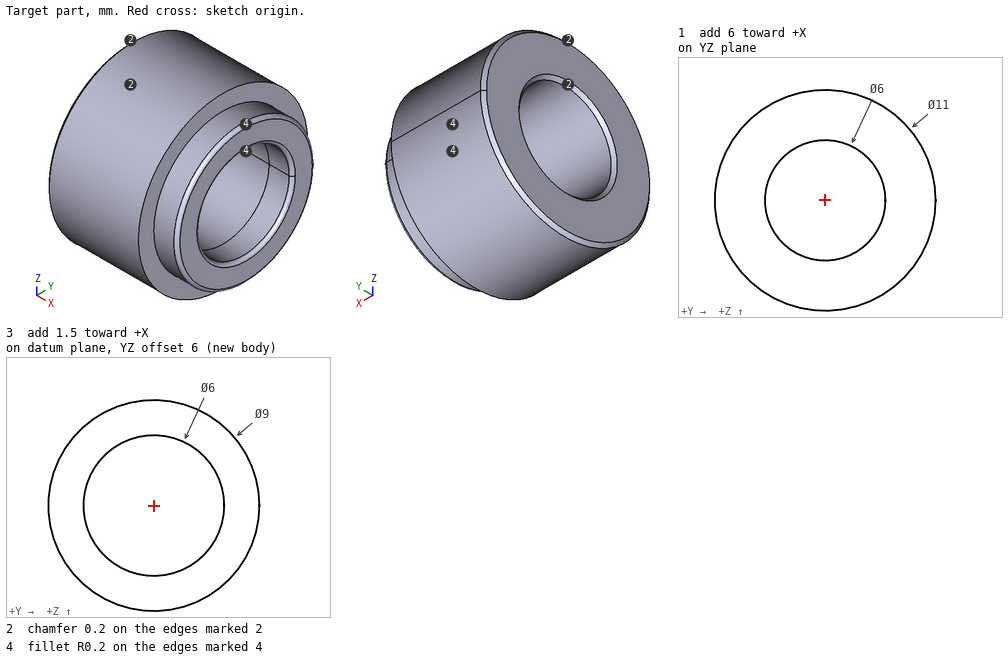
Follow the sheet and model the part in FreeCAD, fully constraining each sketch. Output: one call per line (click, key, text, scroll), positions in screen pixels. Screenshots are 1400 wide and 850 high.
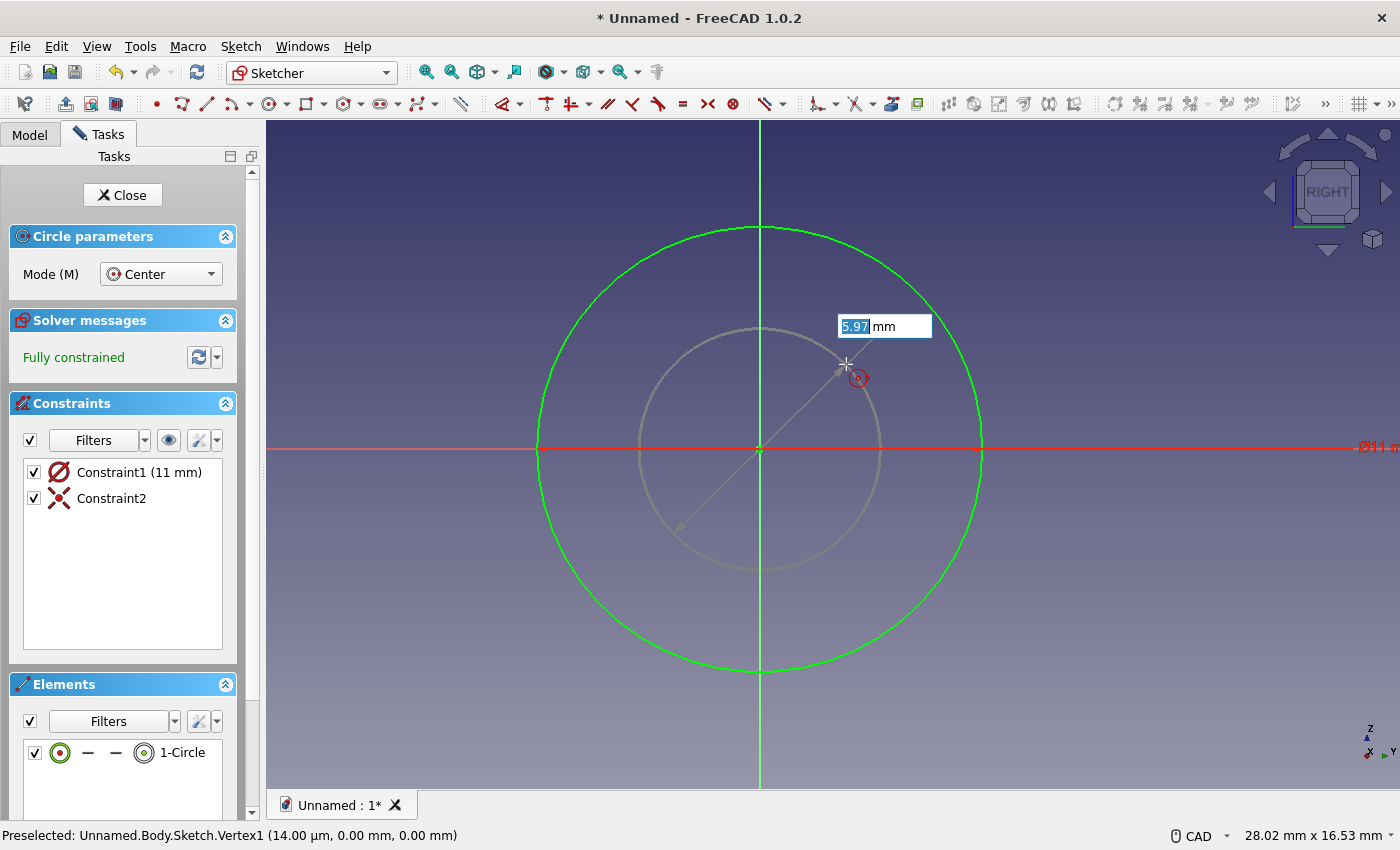
text(6)
key(Return)
key(Escape)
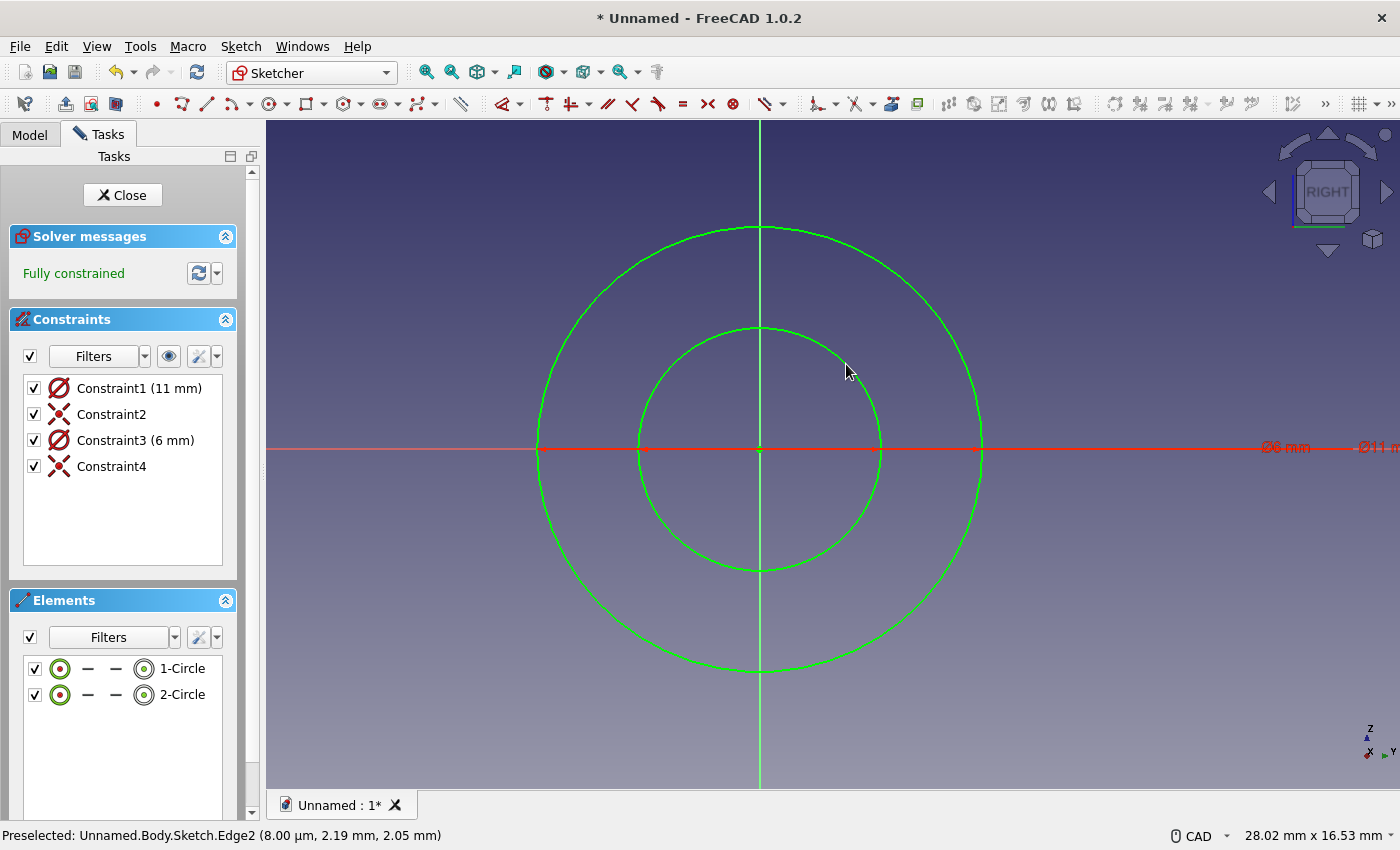
click(123, 195)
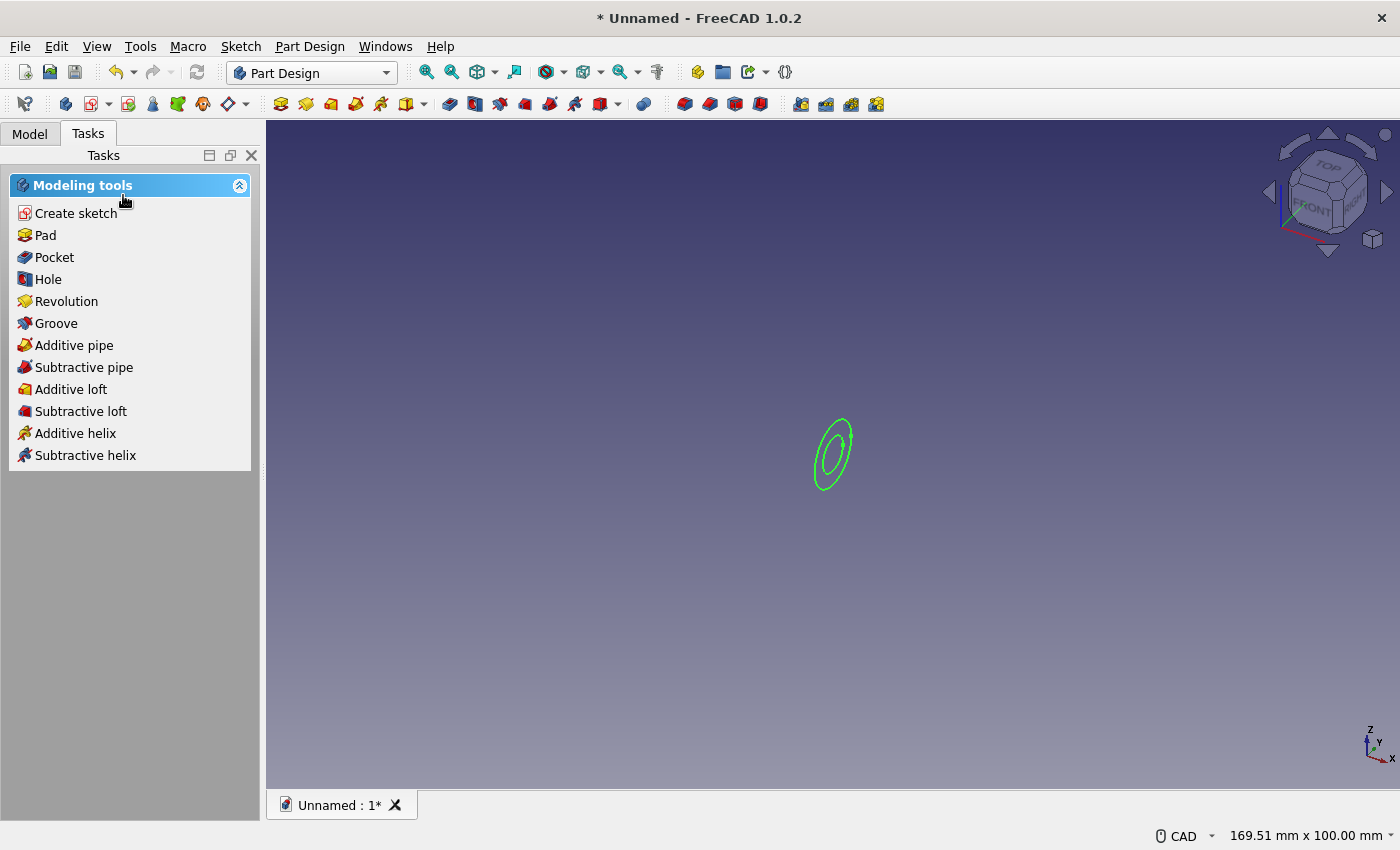
click(281, 104)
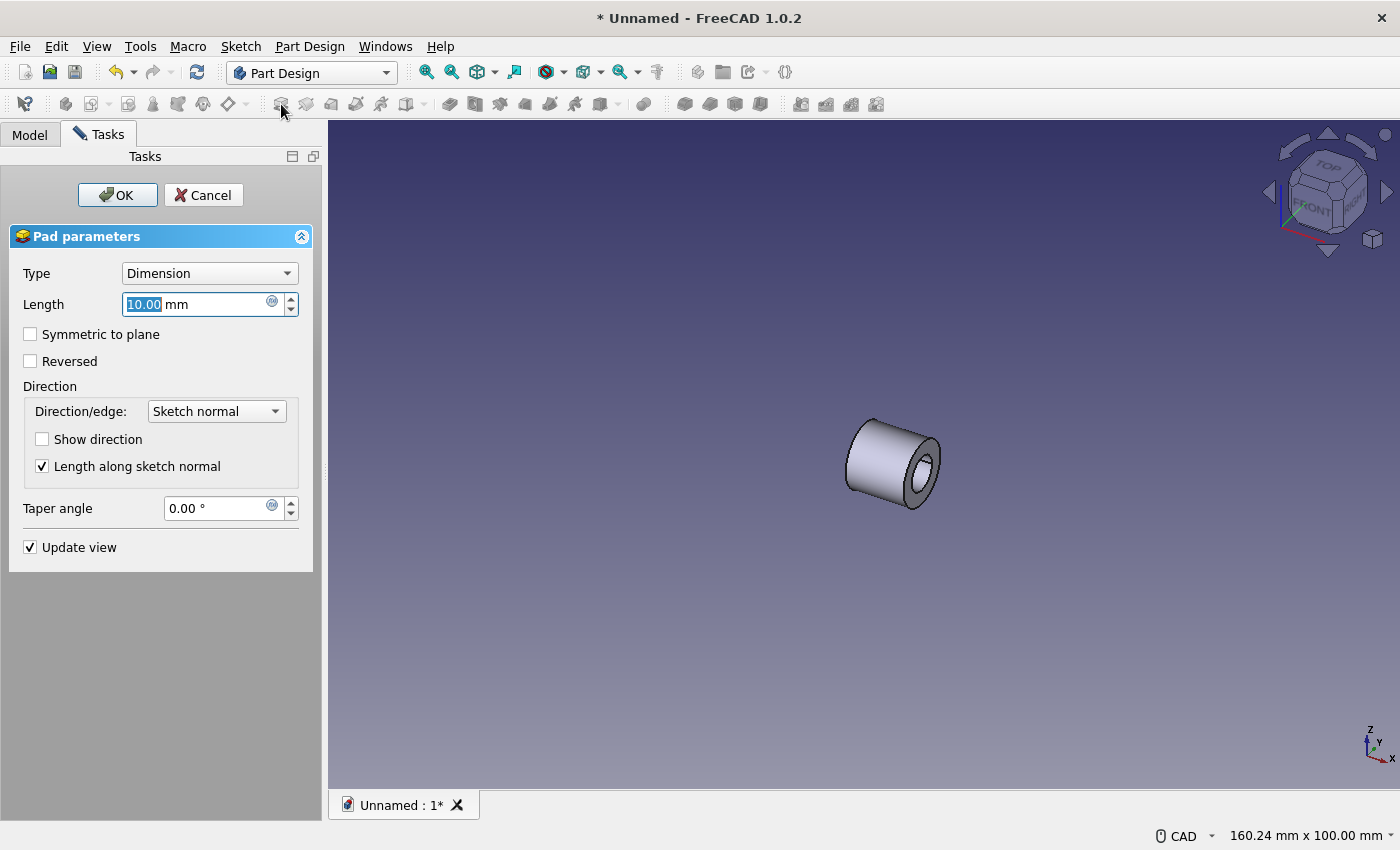
text(6)
key(Tab)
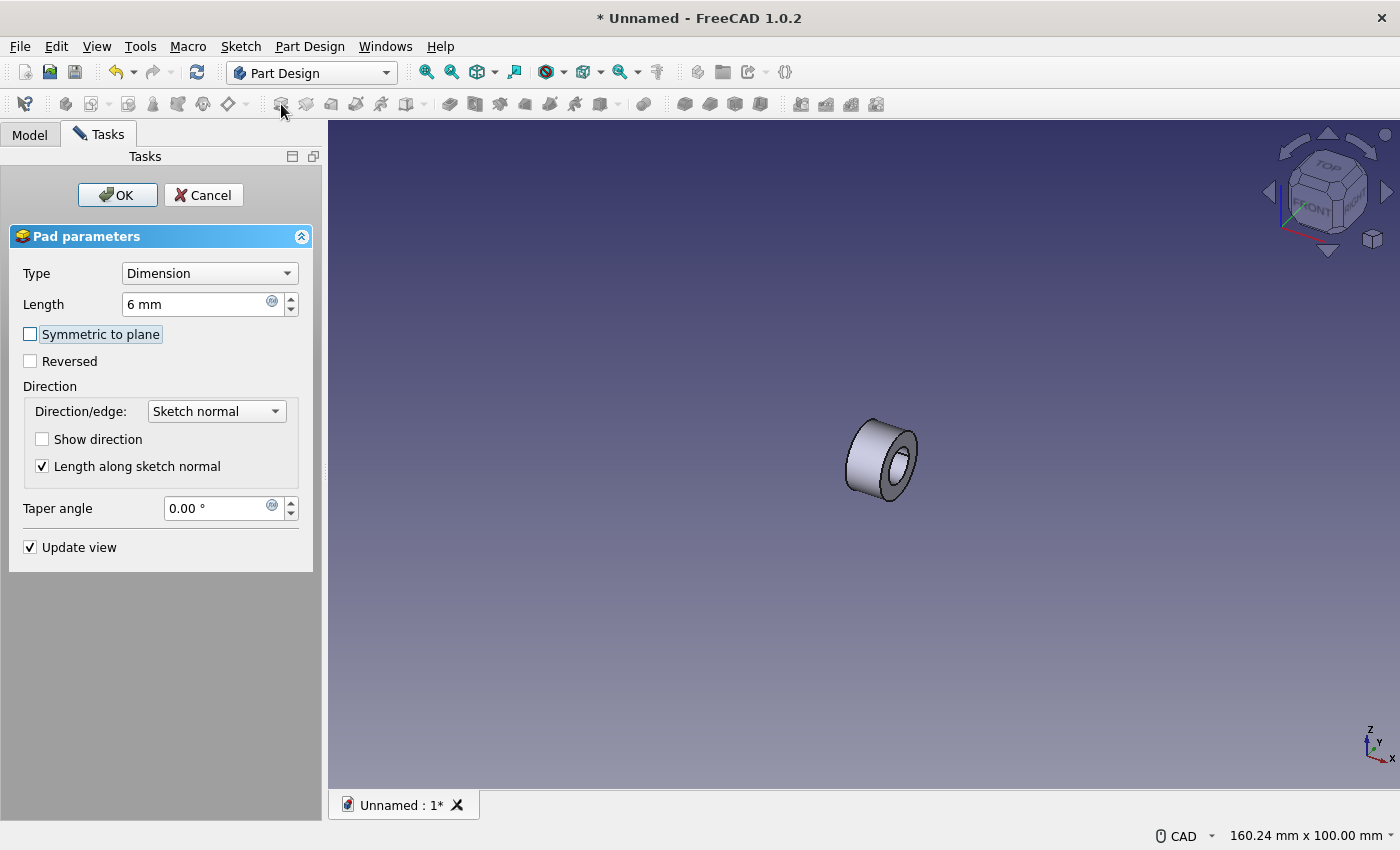
click(118, 195)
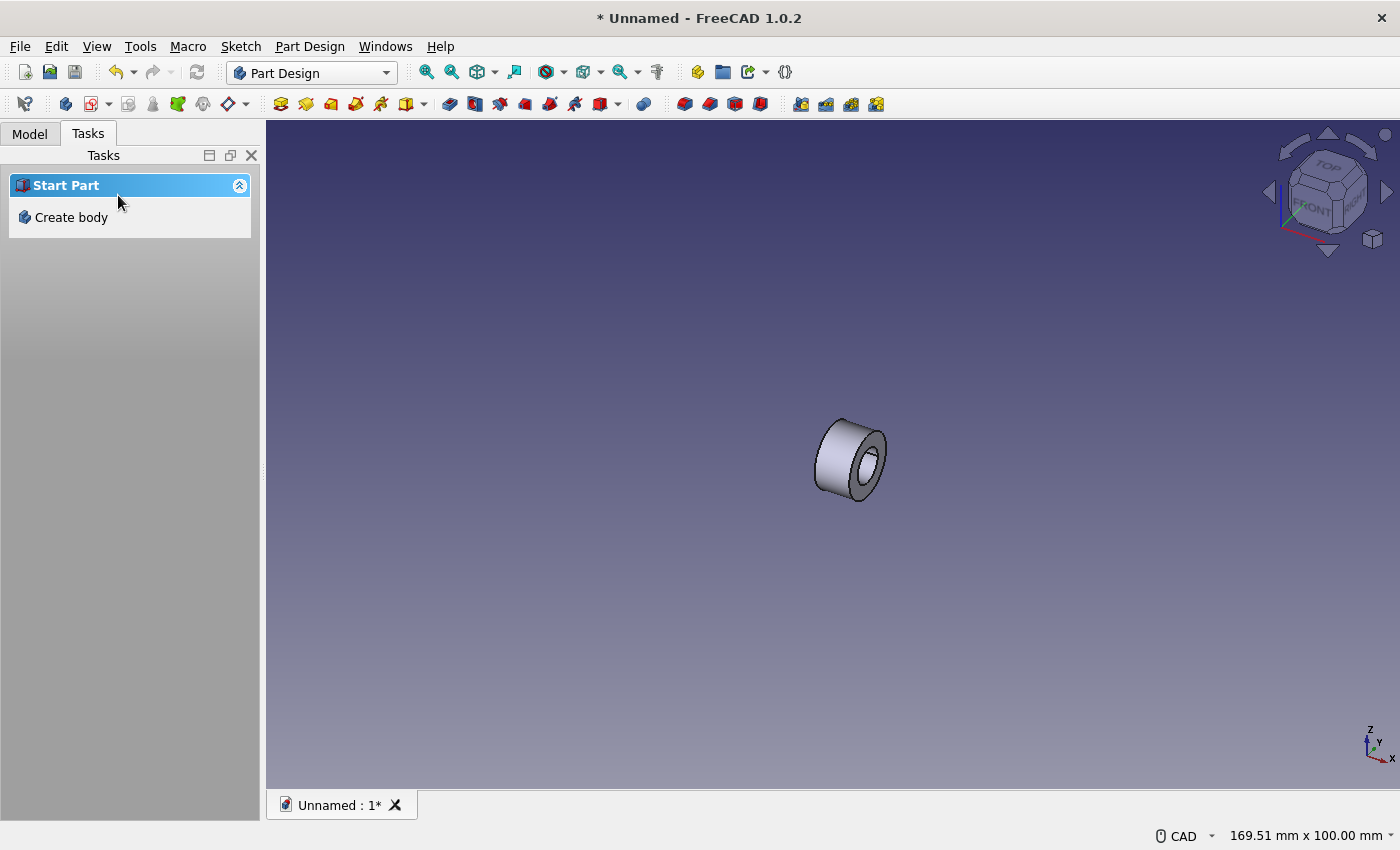
click(427, 72)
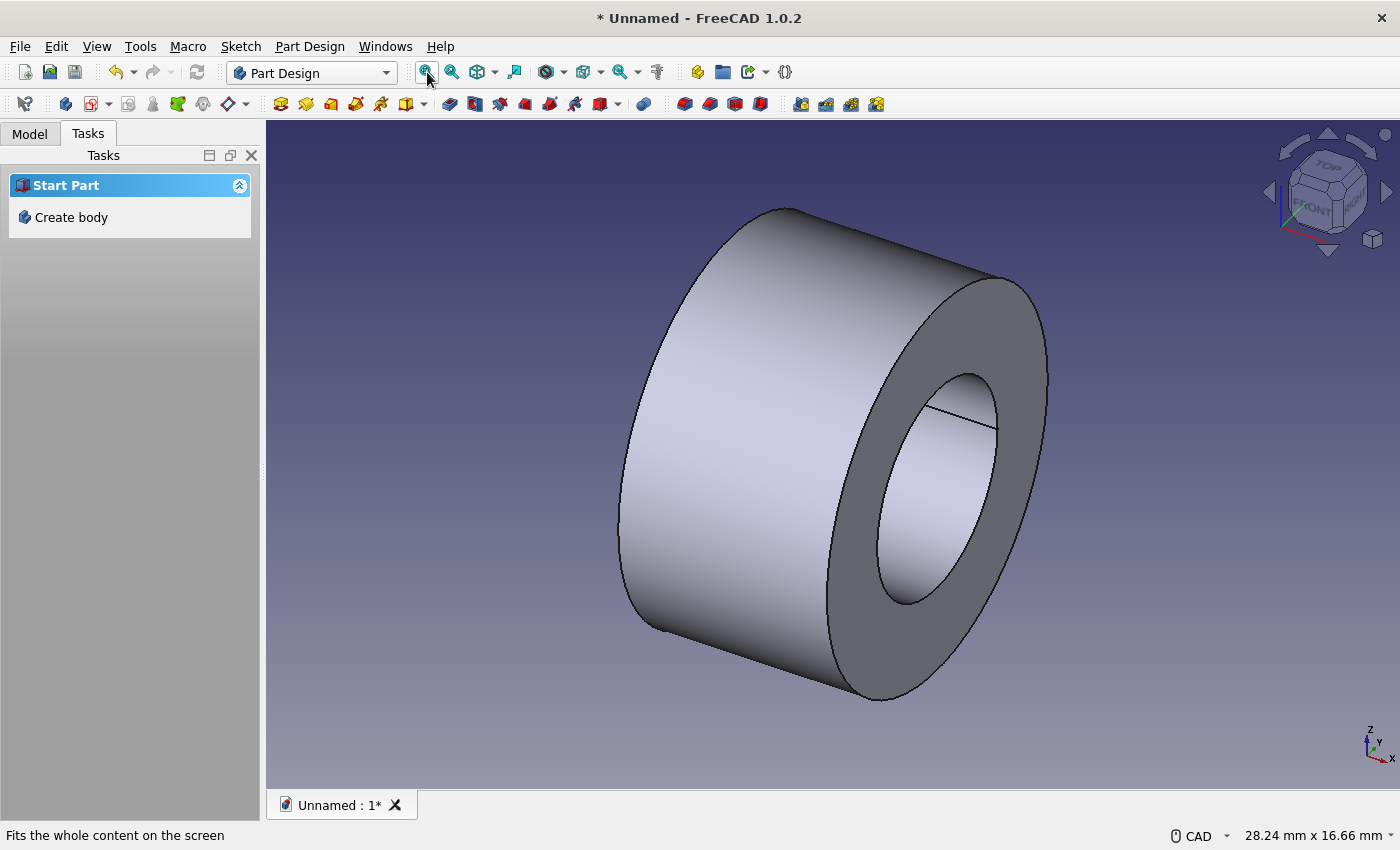
key(0)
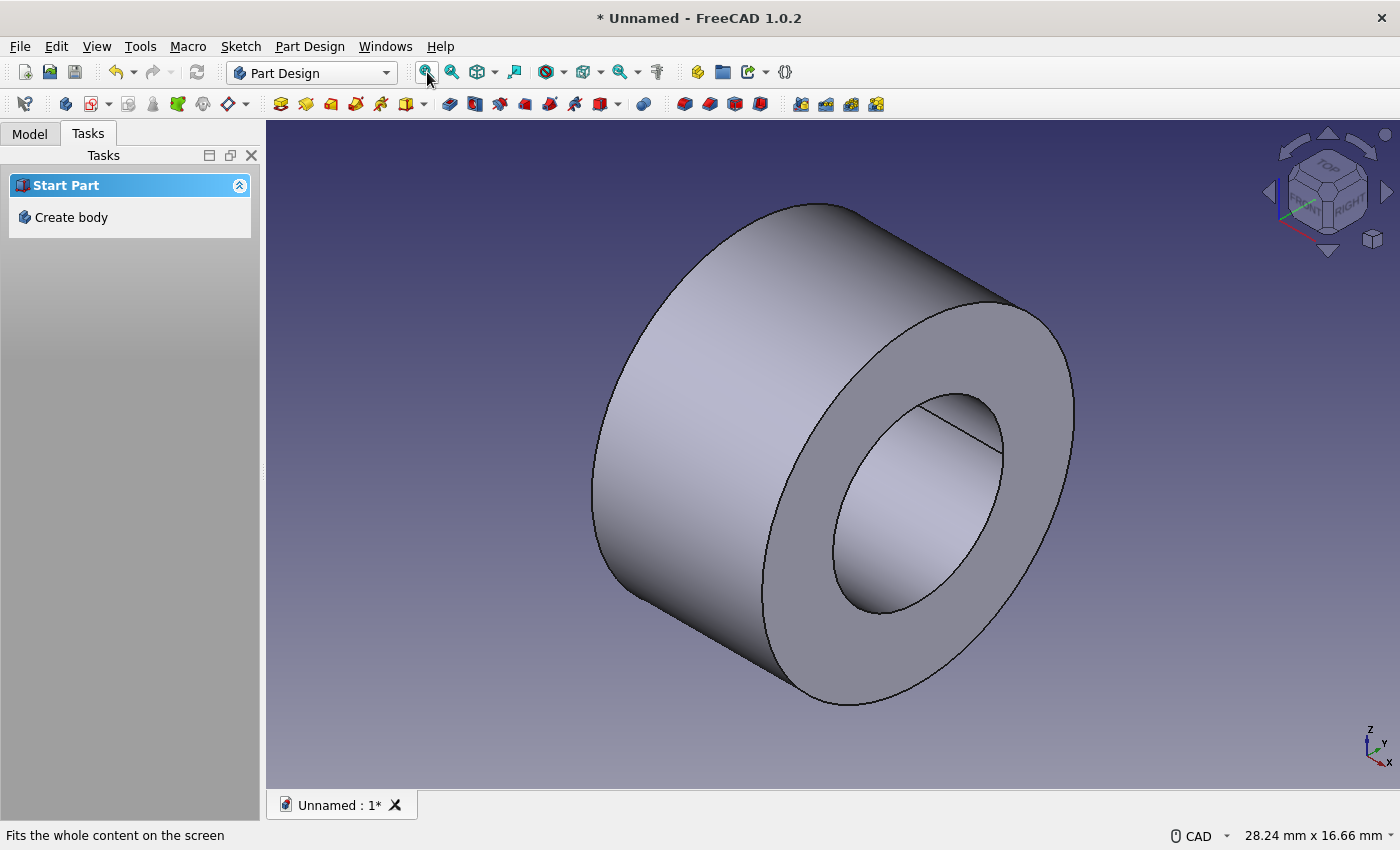
key(2)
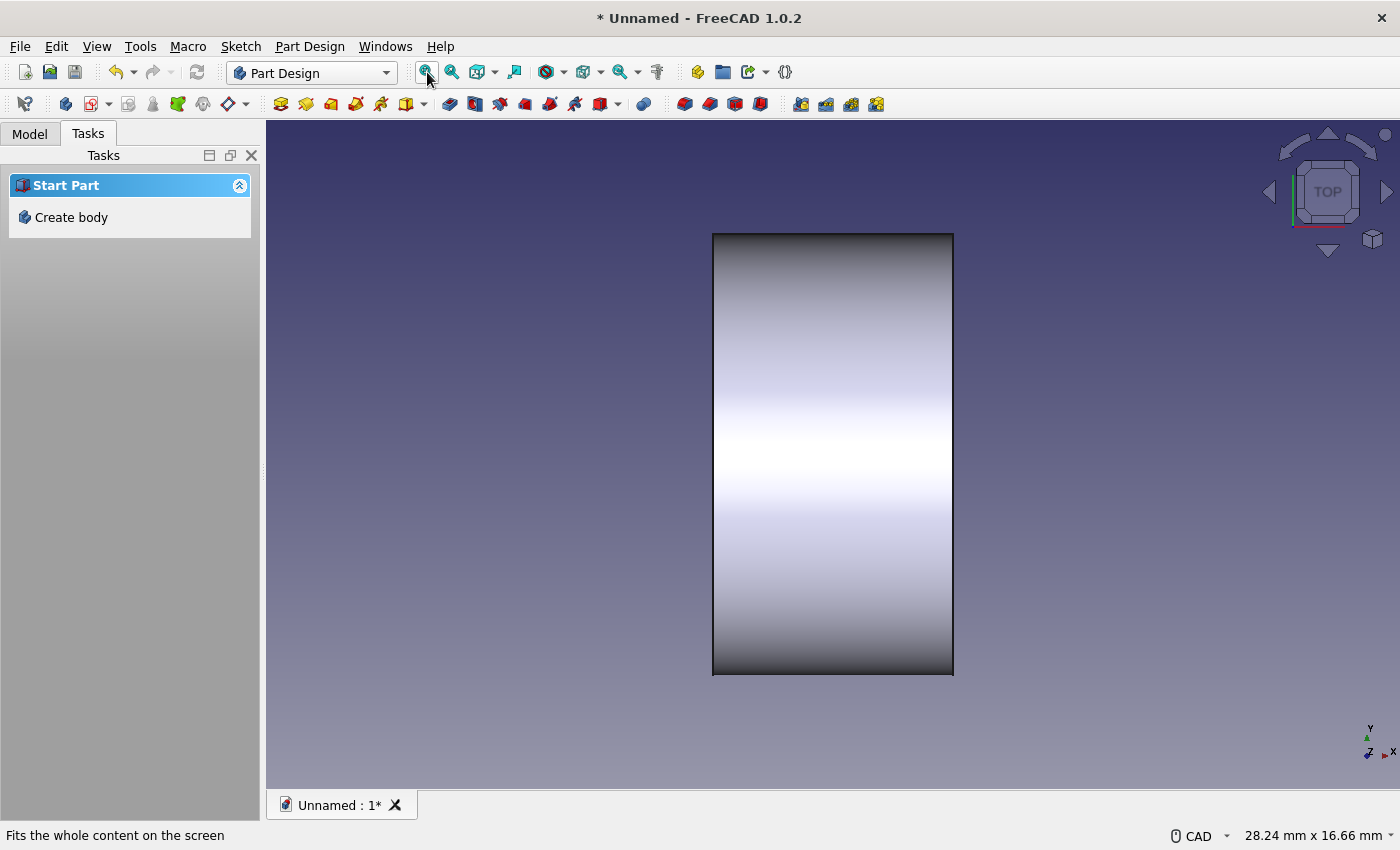
click(713, 632)